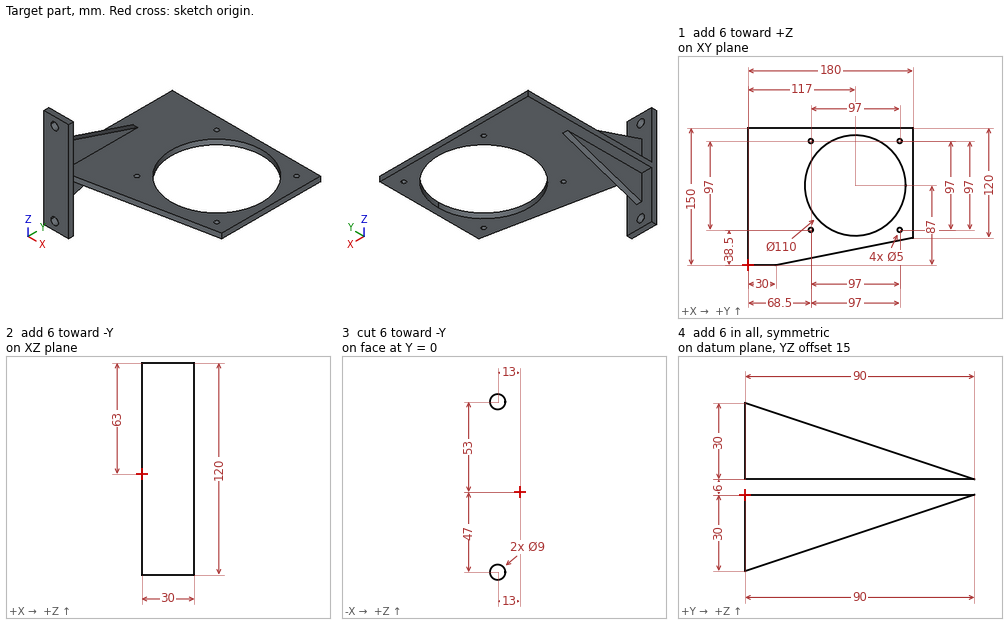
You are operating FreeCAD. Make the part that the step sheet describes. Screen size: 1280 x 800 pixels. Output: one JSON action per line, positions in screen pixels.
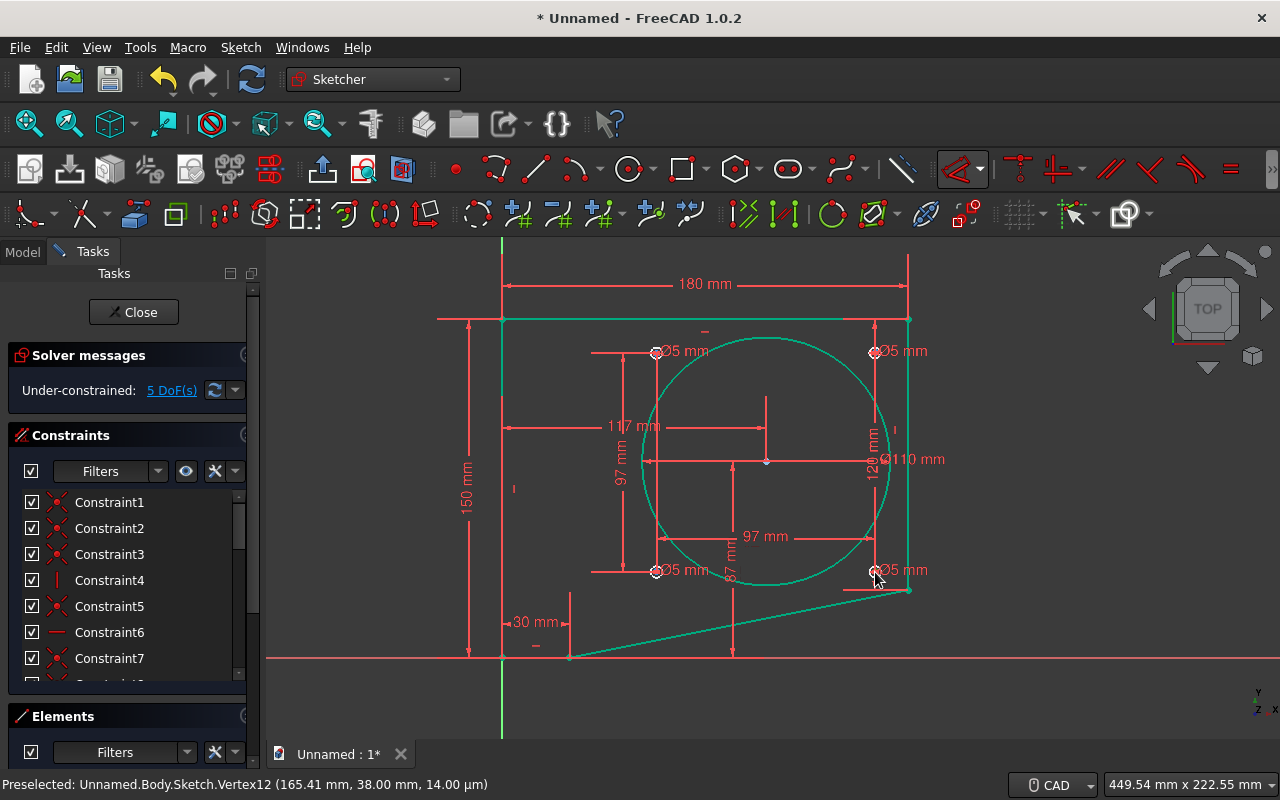
{"action": "left_click", "coordinate": [657, 353]}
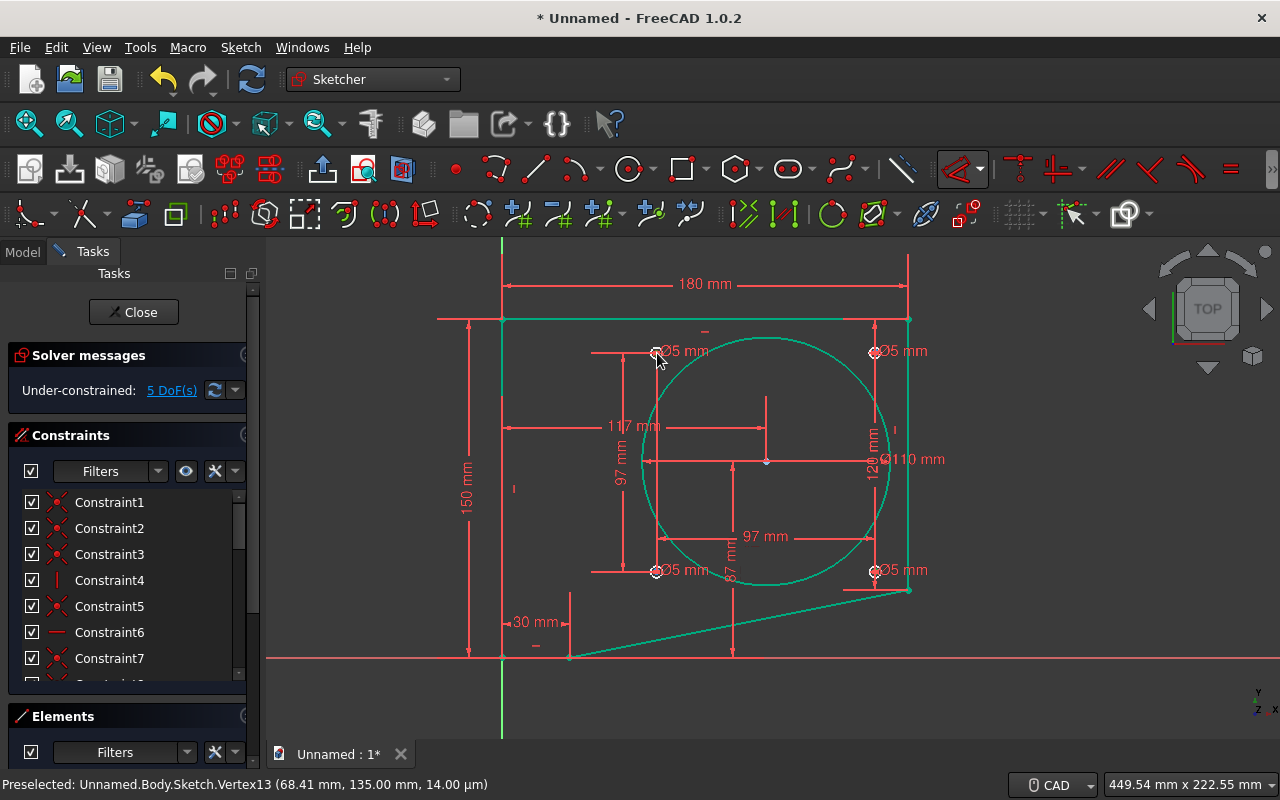
{"action": "key", "text": "i"}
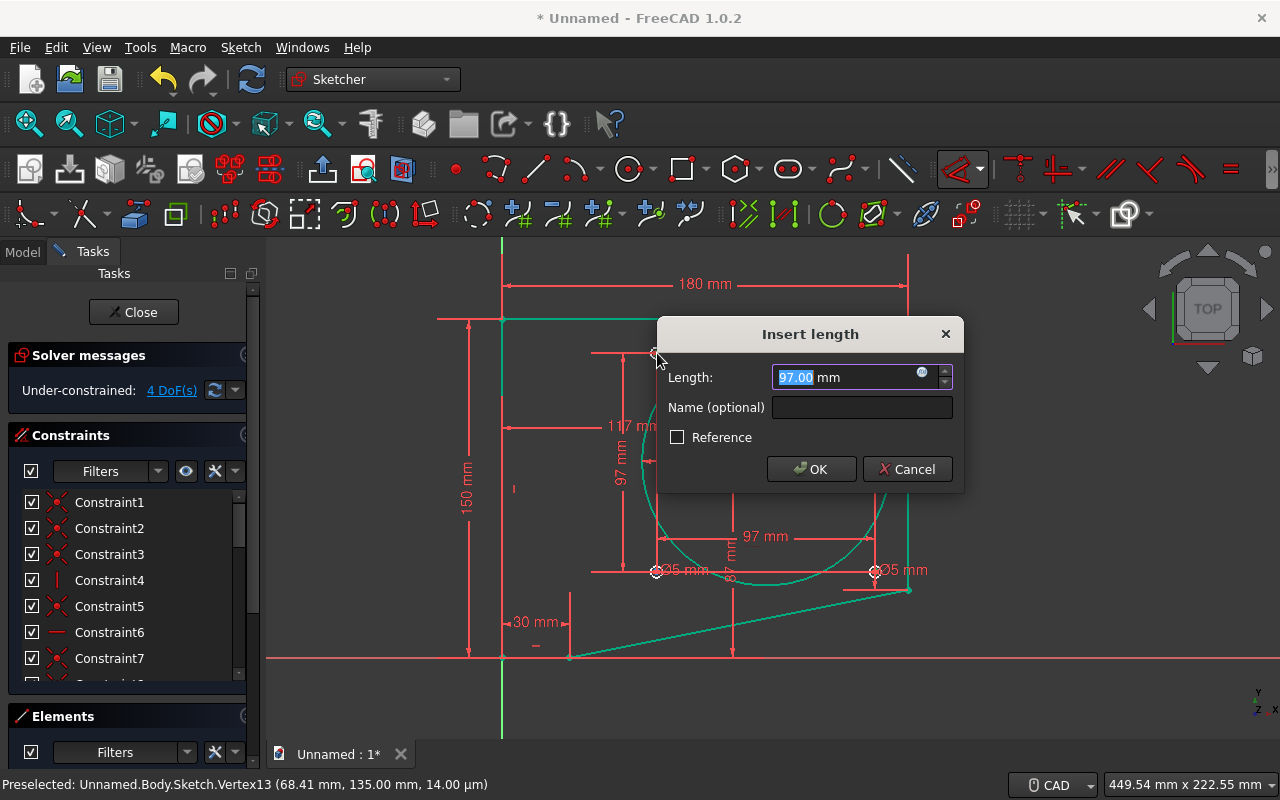
{"action": "type", "text": "97"}
{"action": "key", "text": "Return"}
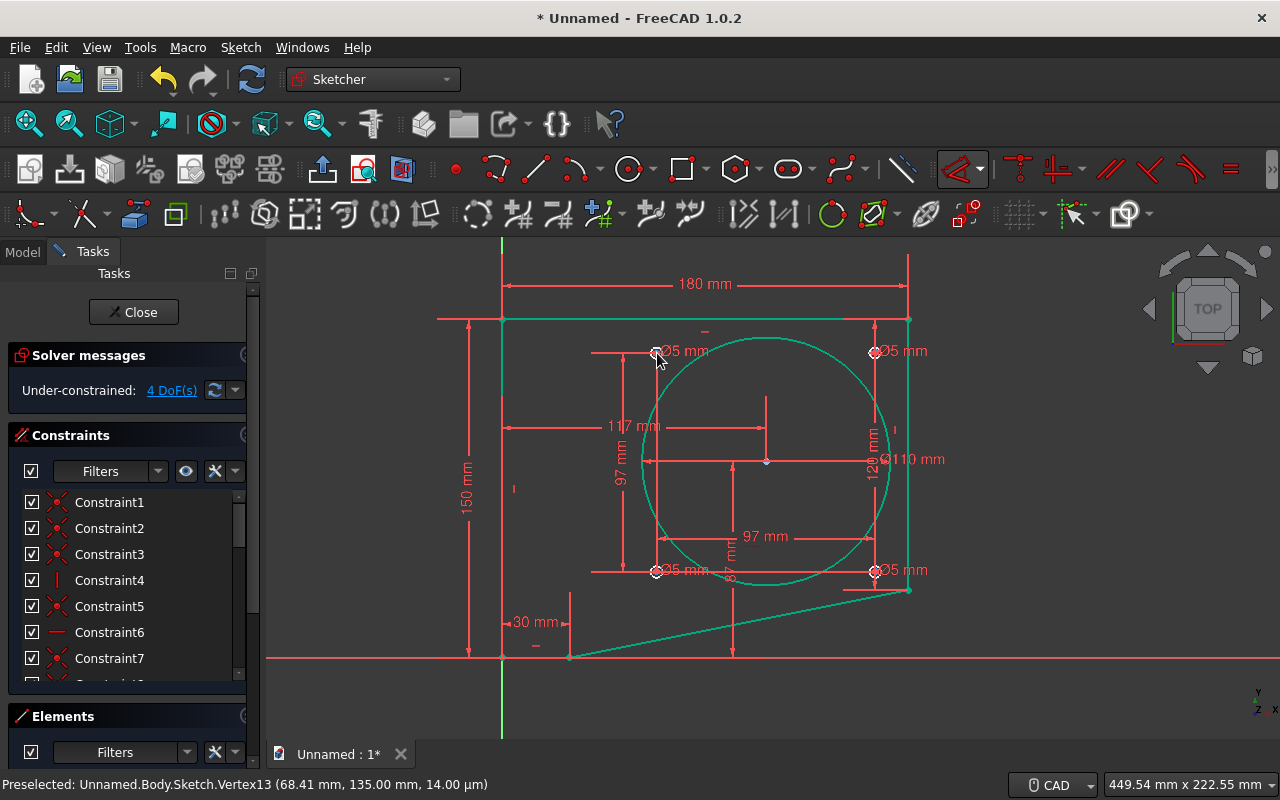
{"action": "left_click", "coordinate": [657, 353]}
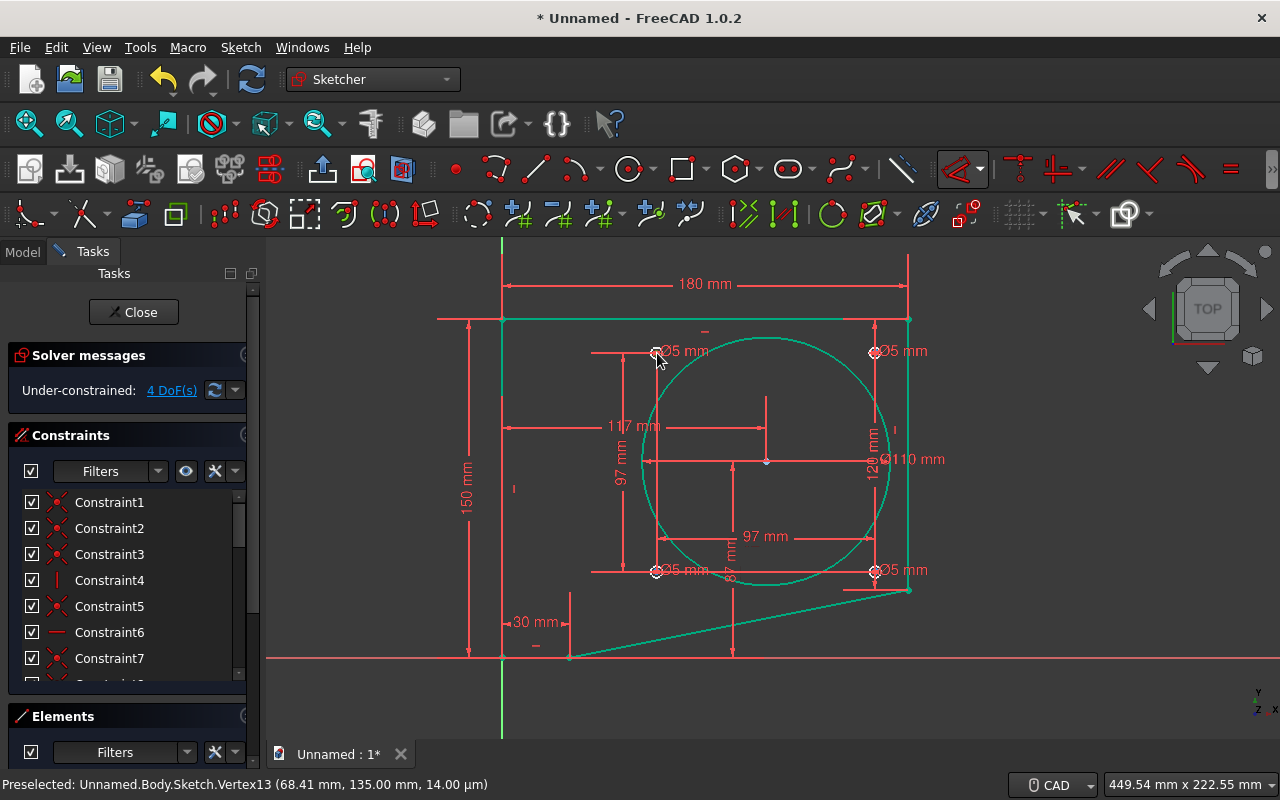
{"action": "left_click", "coordinate": [875, 353]}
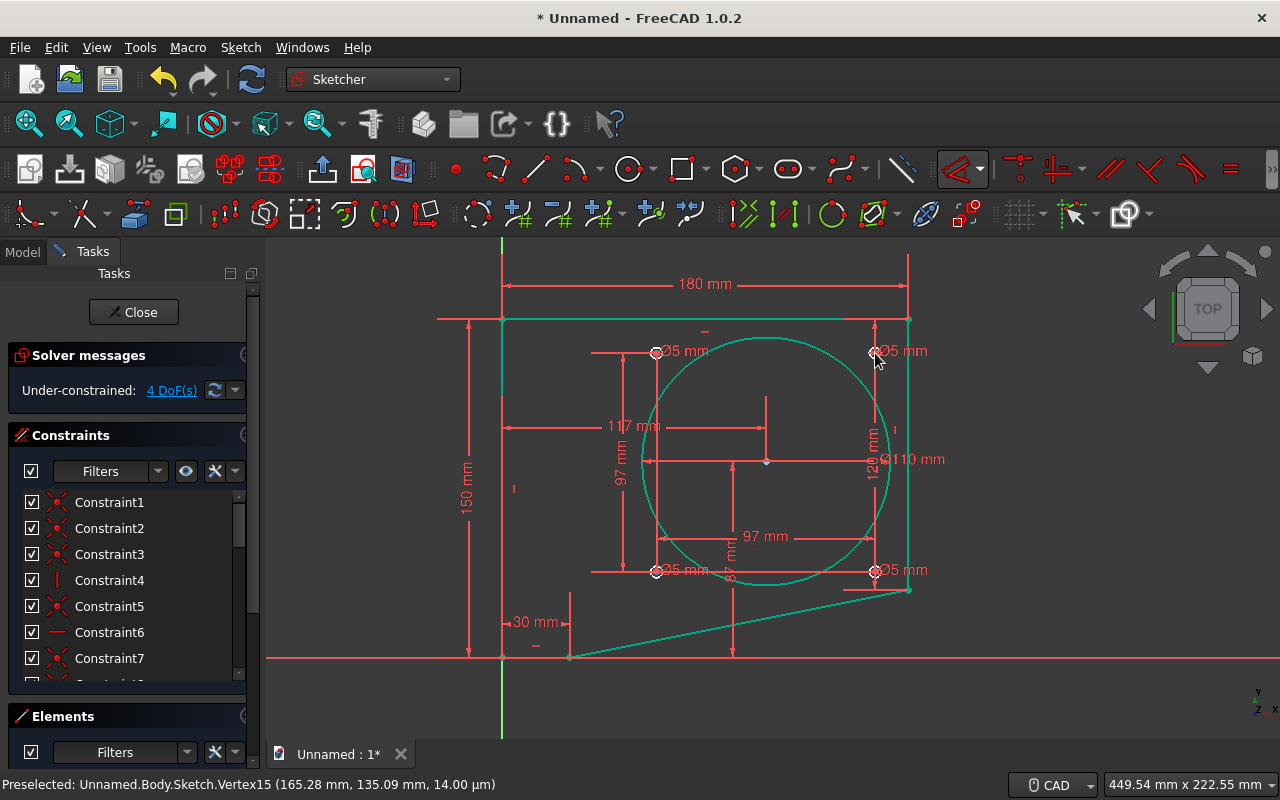
{"action": "left_click", "coordinate": [982, 170]}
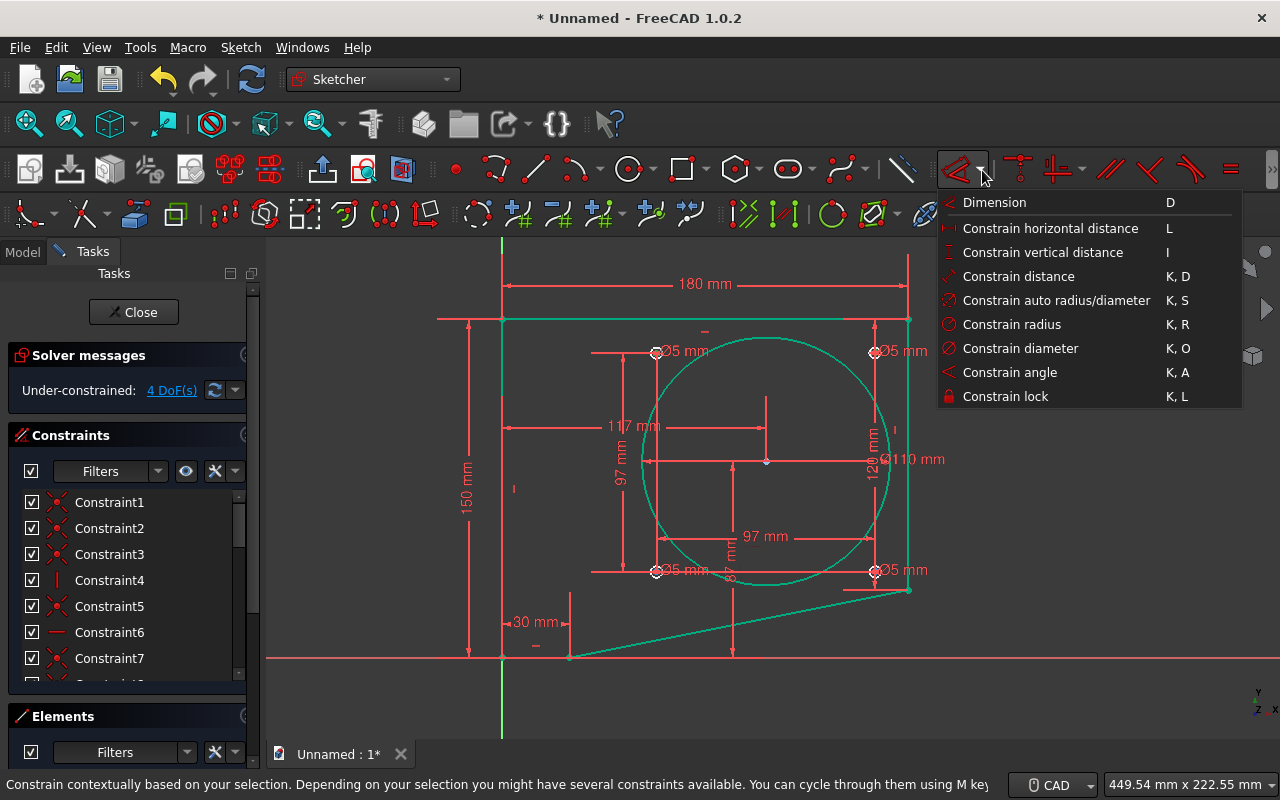
{"action": "left_click", "coordinate": [1090, 228]}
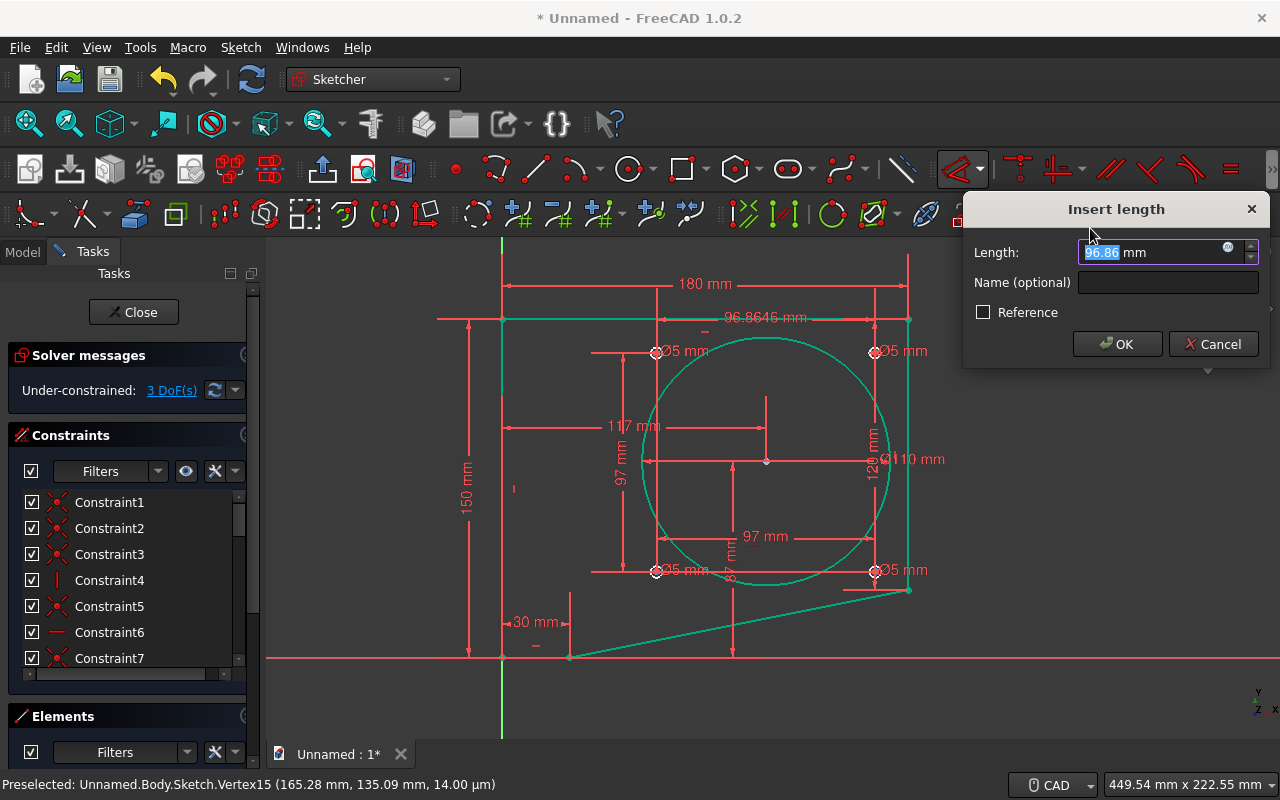
{"action": "type", "text": "97"}
{"action": "key", "text": "Return"}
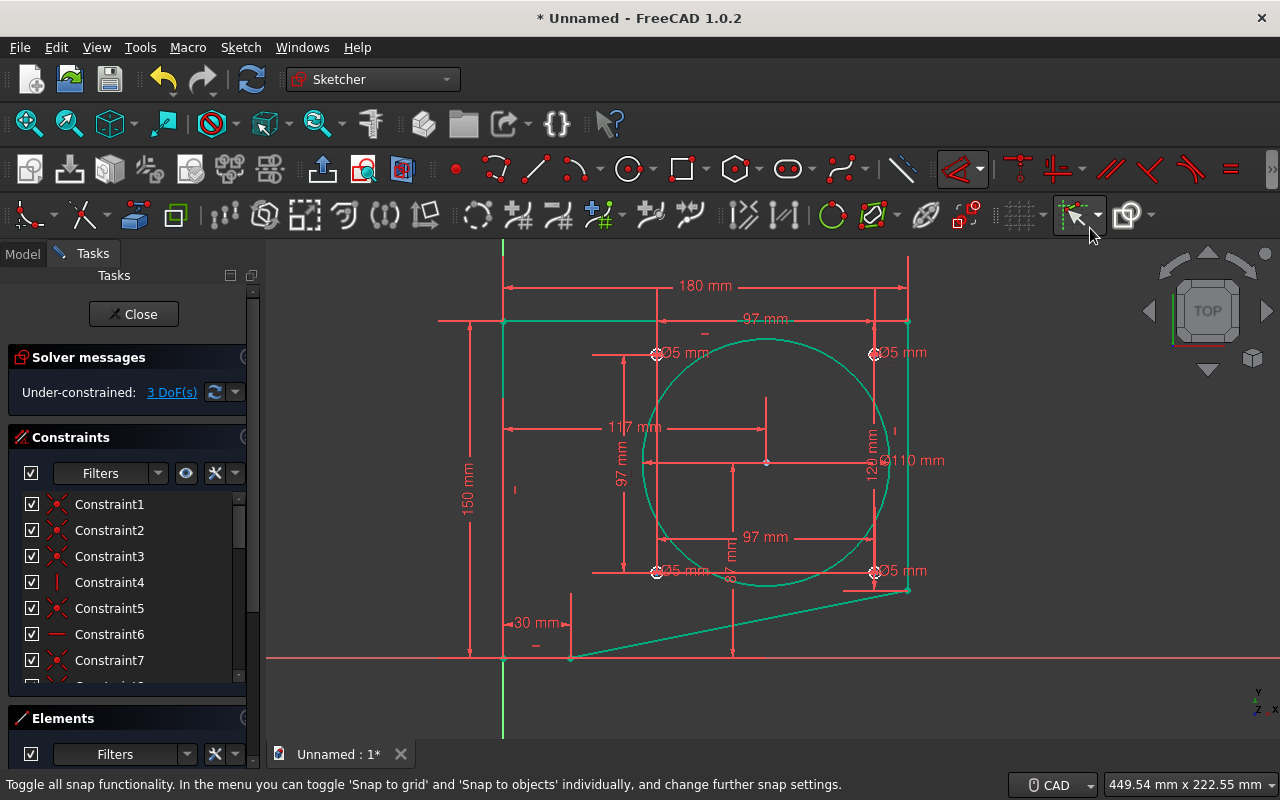
{"action": "left_click", "coordinate": [875, 573]}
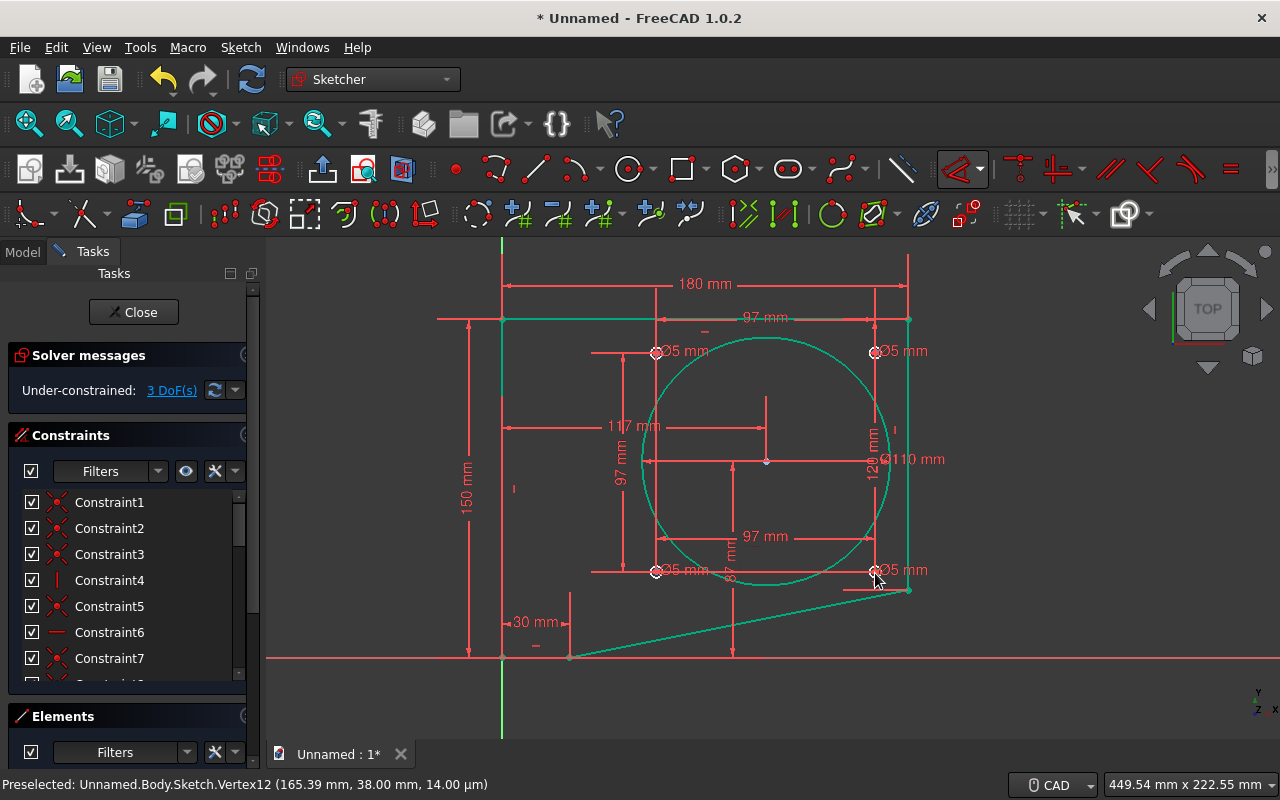
{"action": "left_click", "coordinate": [875, 353]}